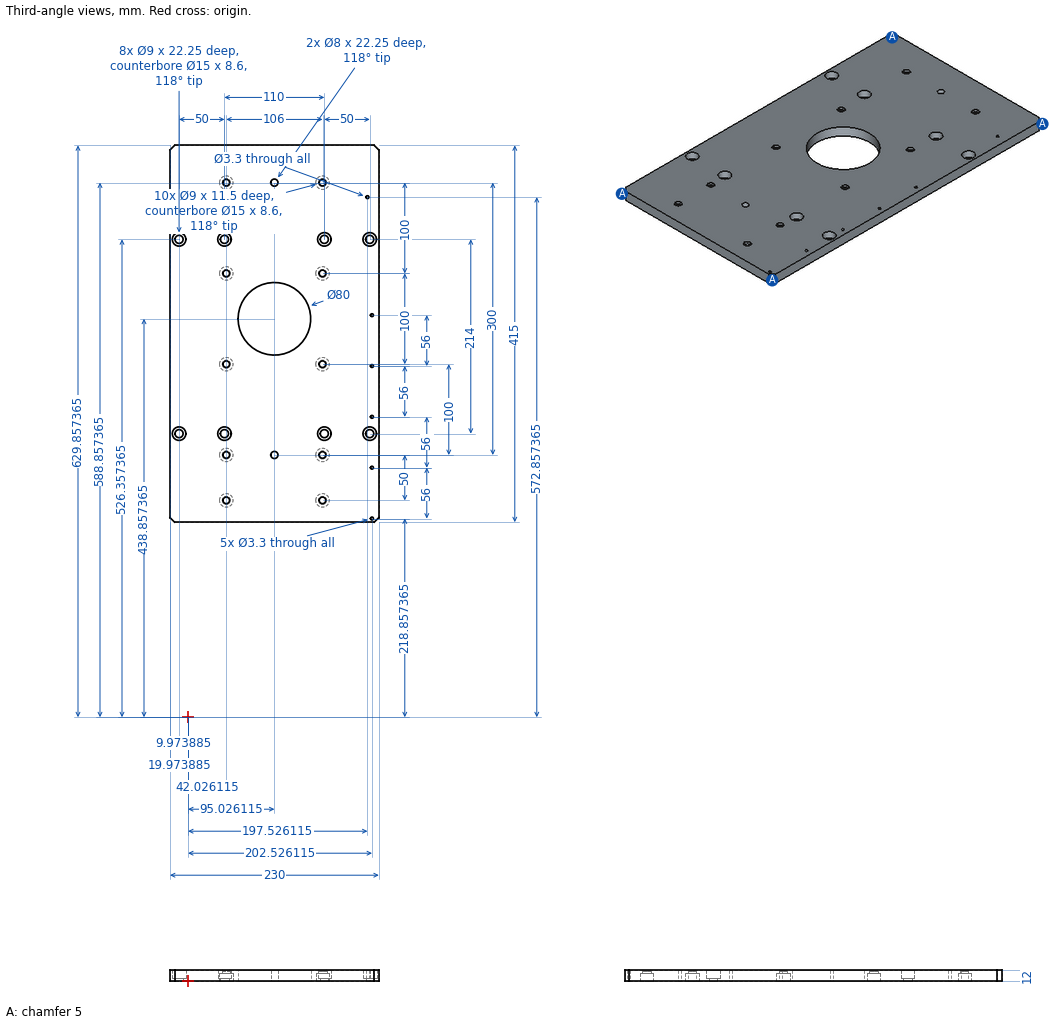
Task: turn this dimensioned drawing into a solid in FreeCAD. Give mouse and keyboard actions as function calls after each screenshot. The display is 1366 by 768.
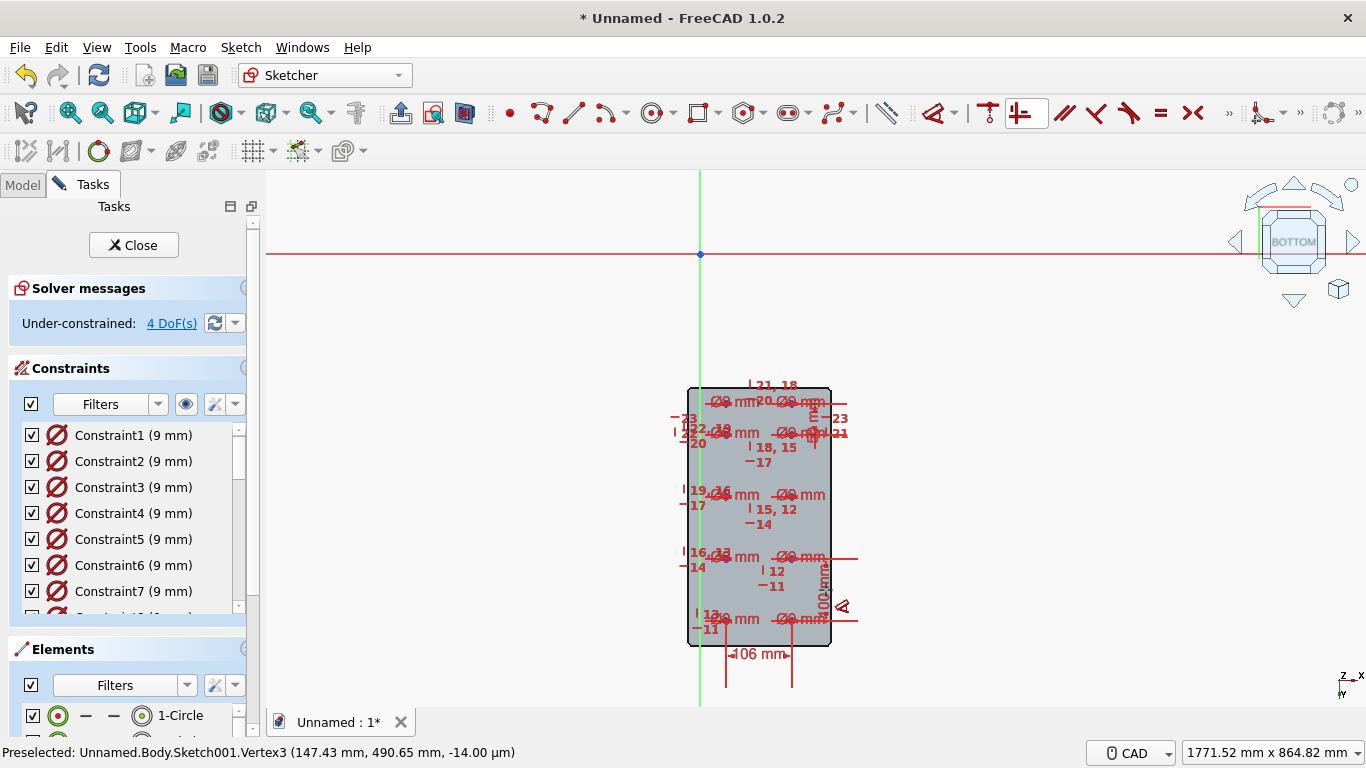
click(792, 559)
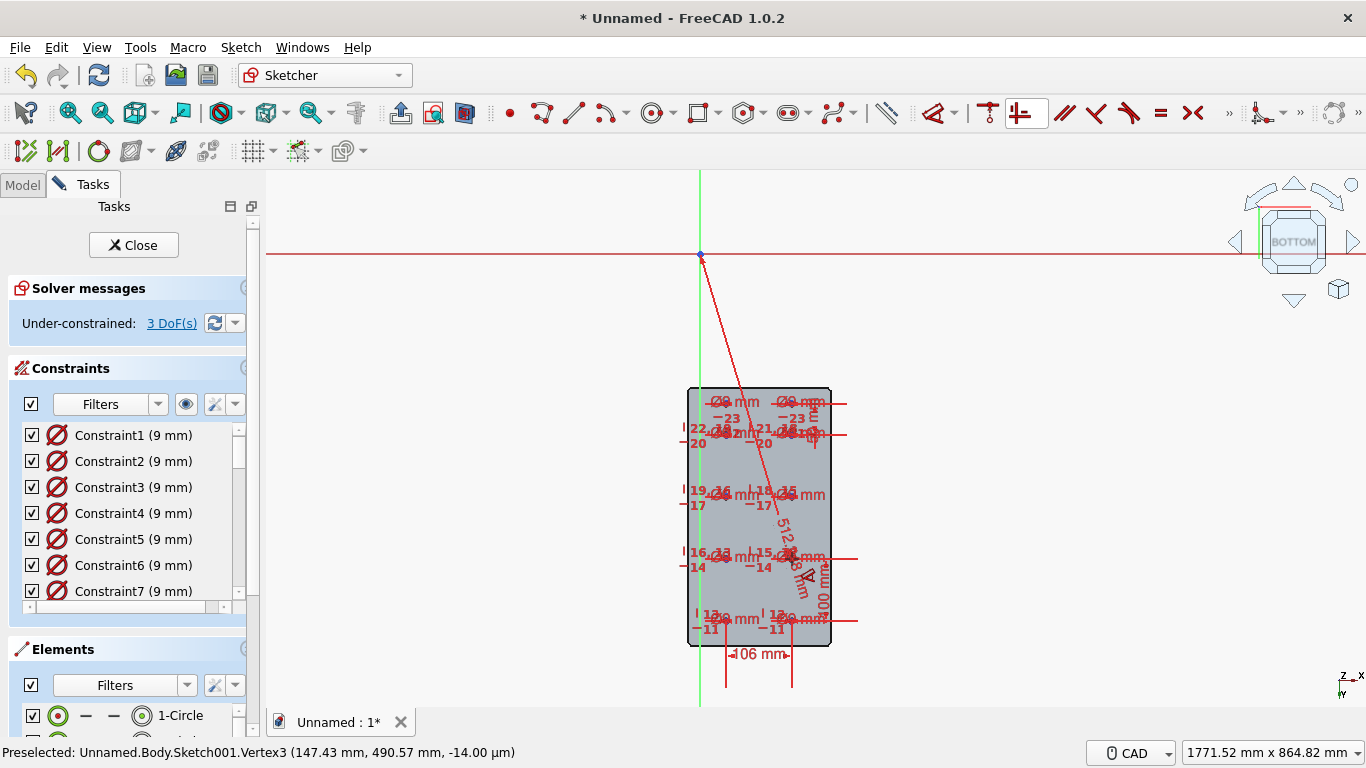
click(792, 497)
click(826, 528)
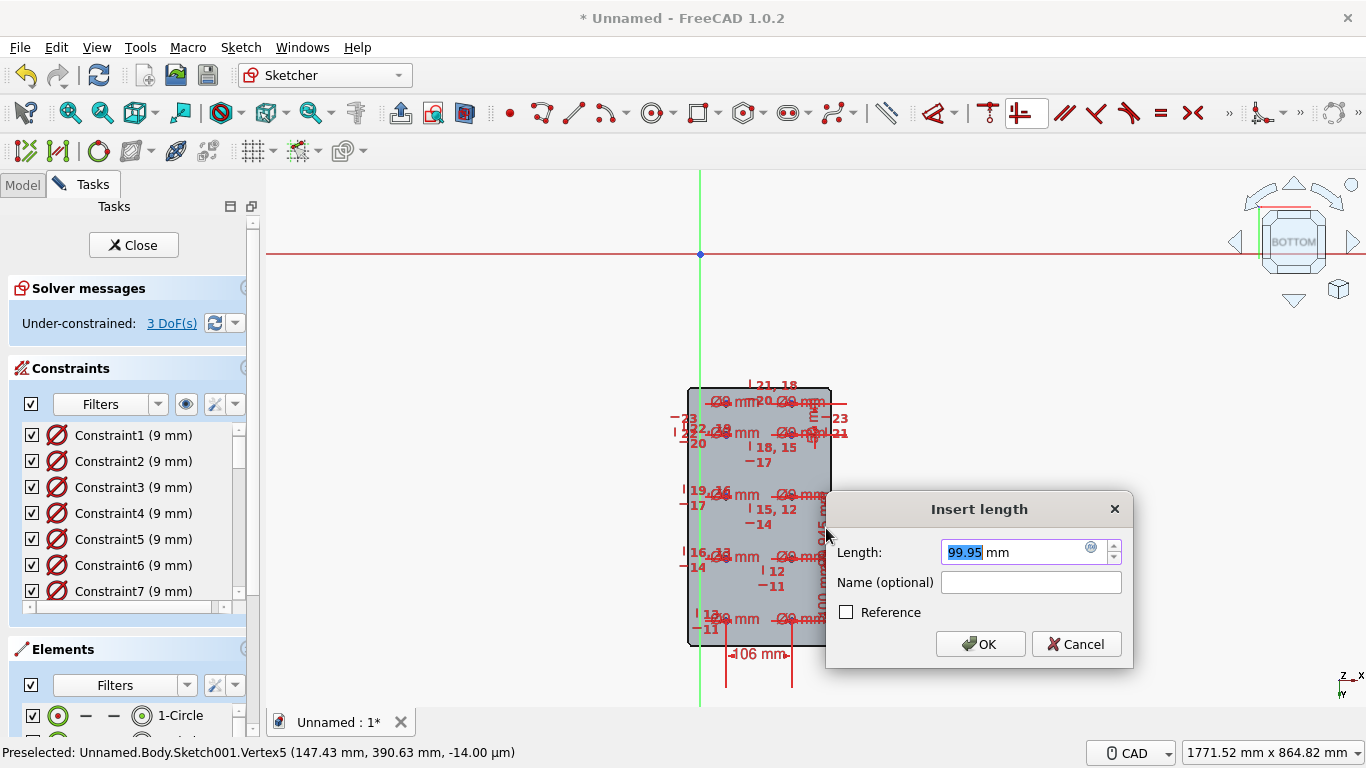
text(100)
key(Return)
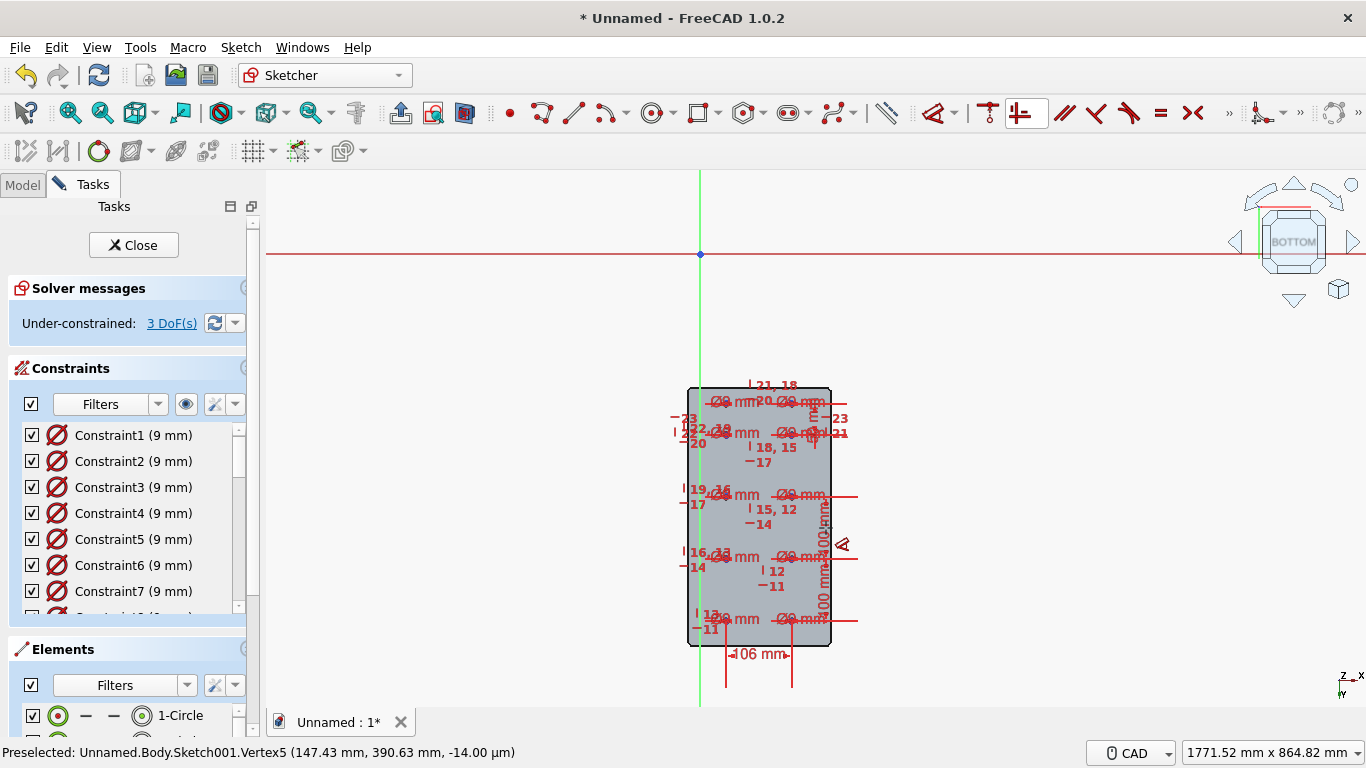
click(792, 497)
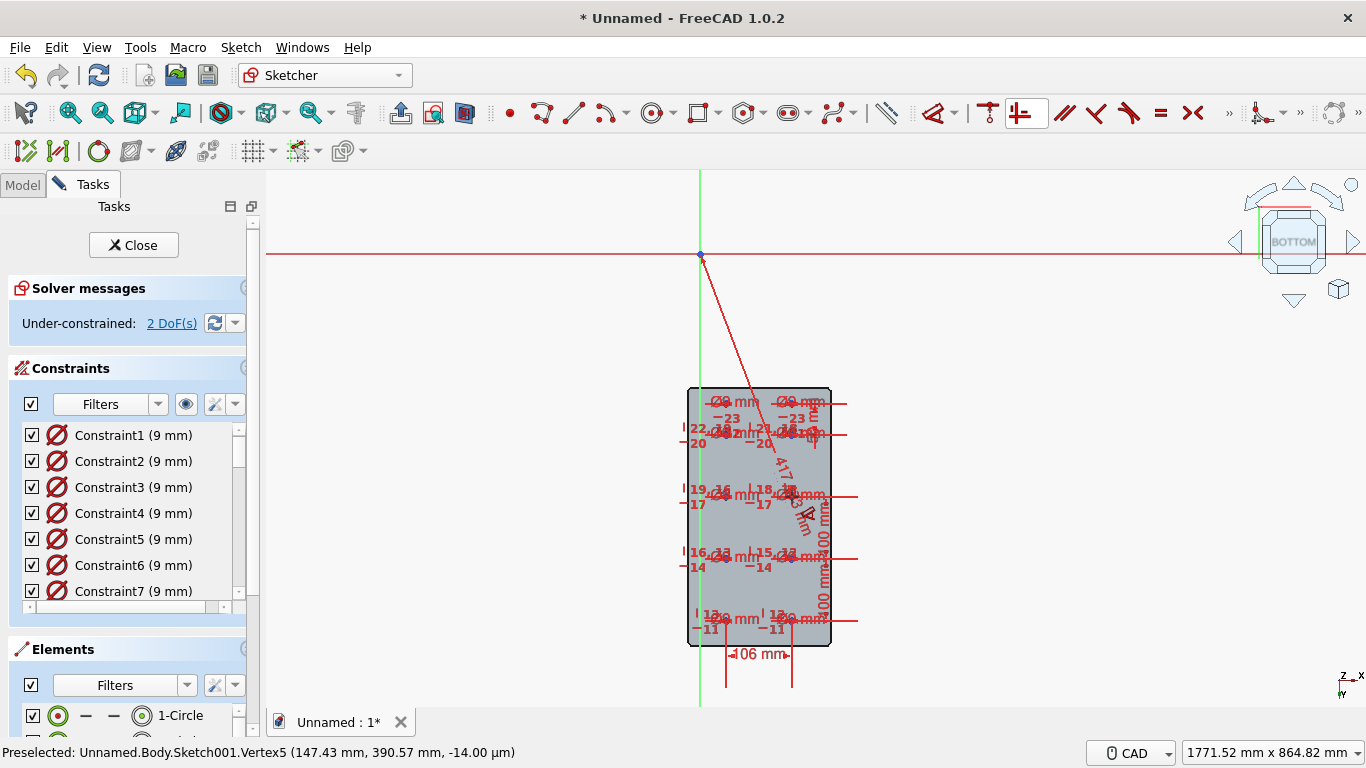
click(792, 435)
click(826, 466)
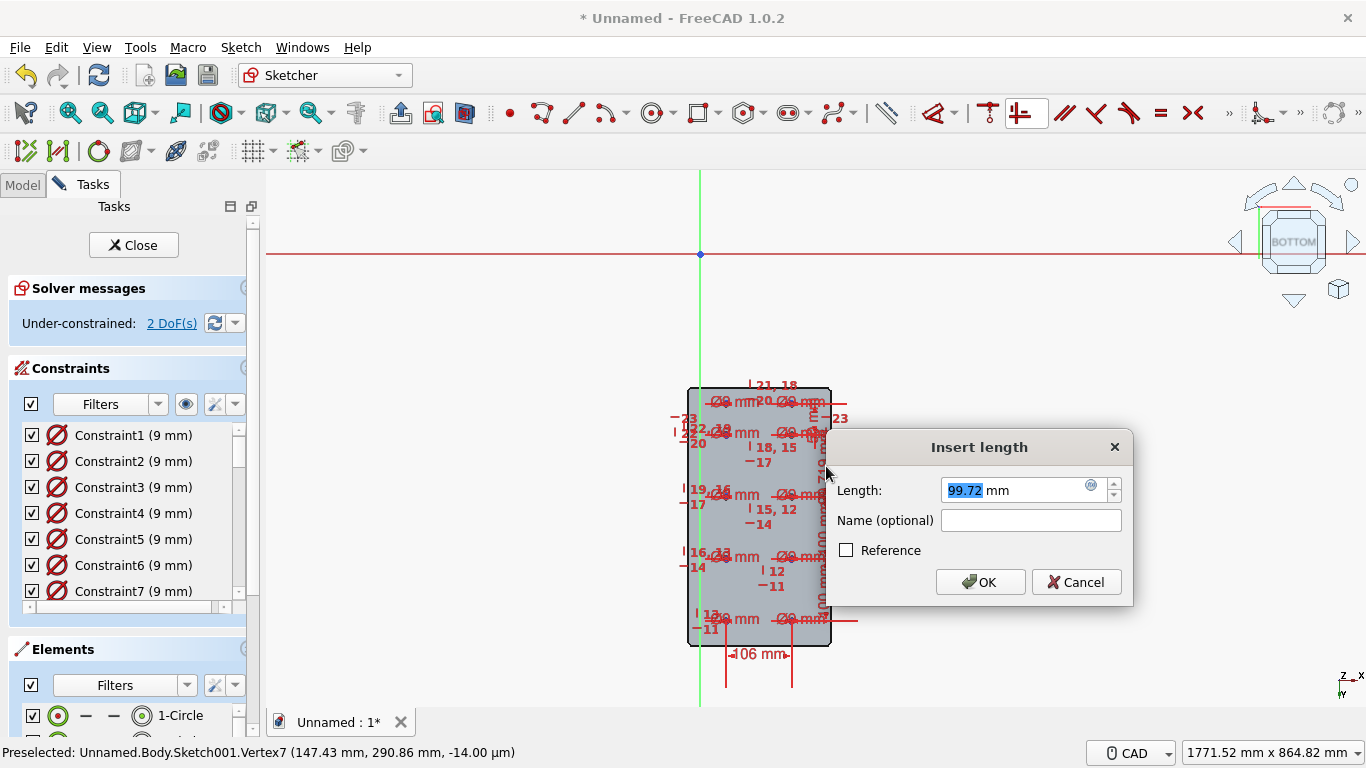
text(100)
key(Return)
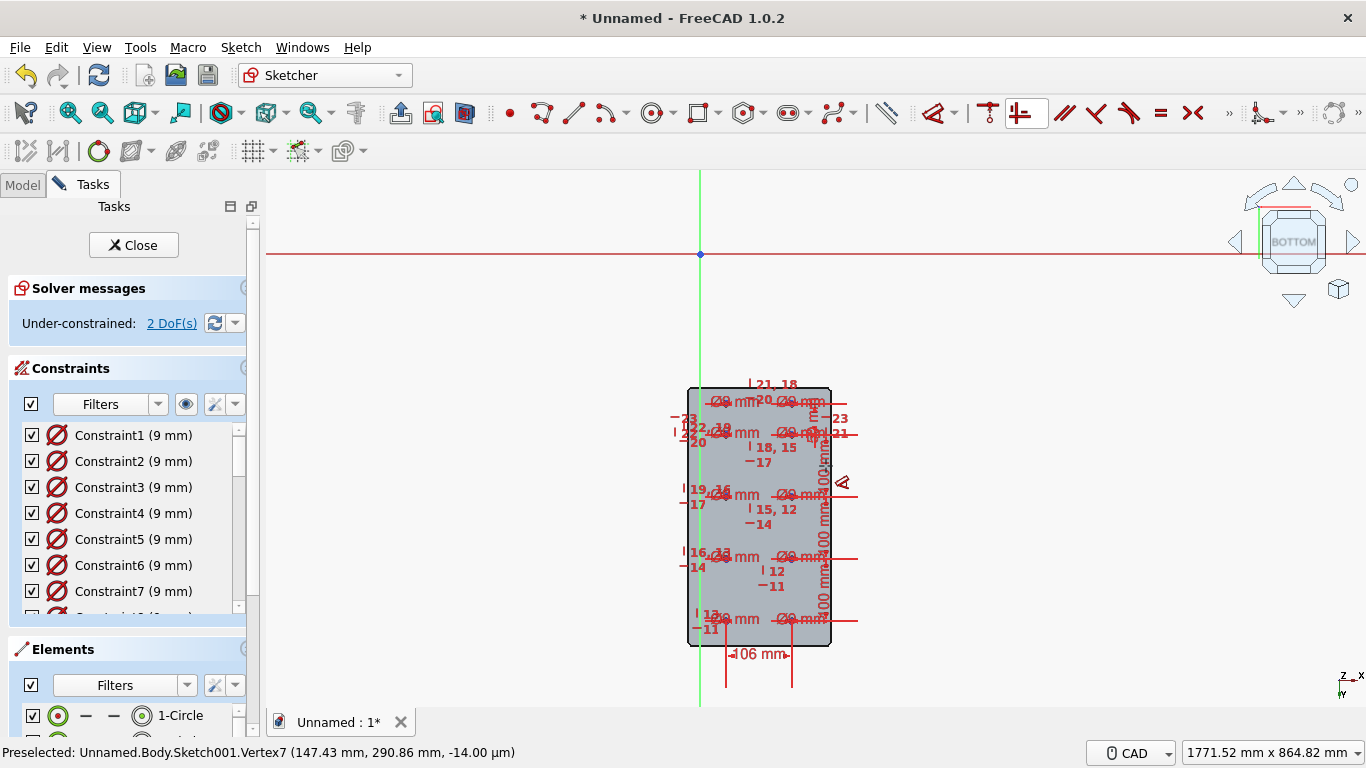
scroll(726, 621, up, 3)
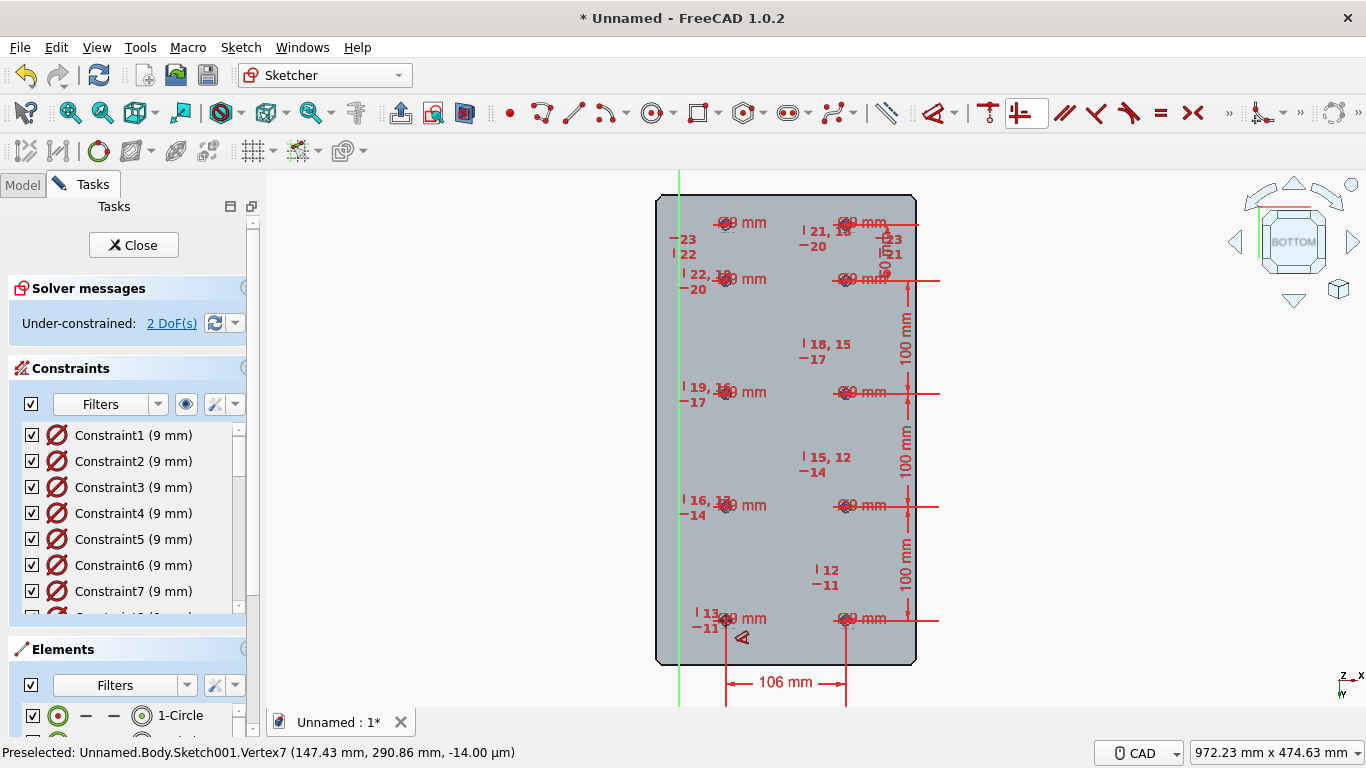
click(726, 621)
click(702, 655)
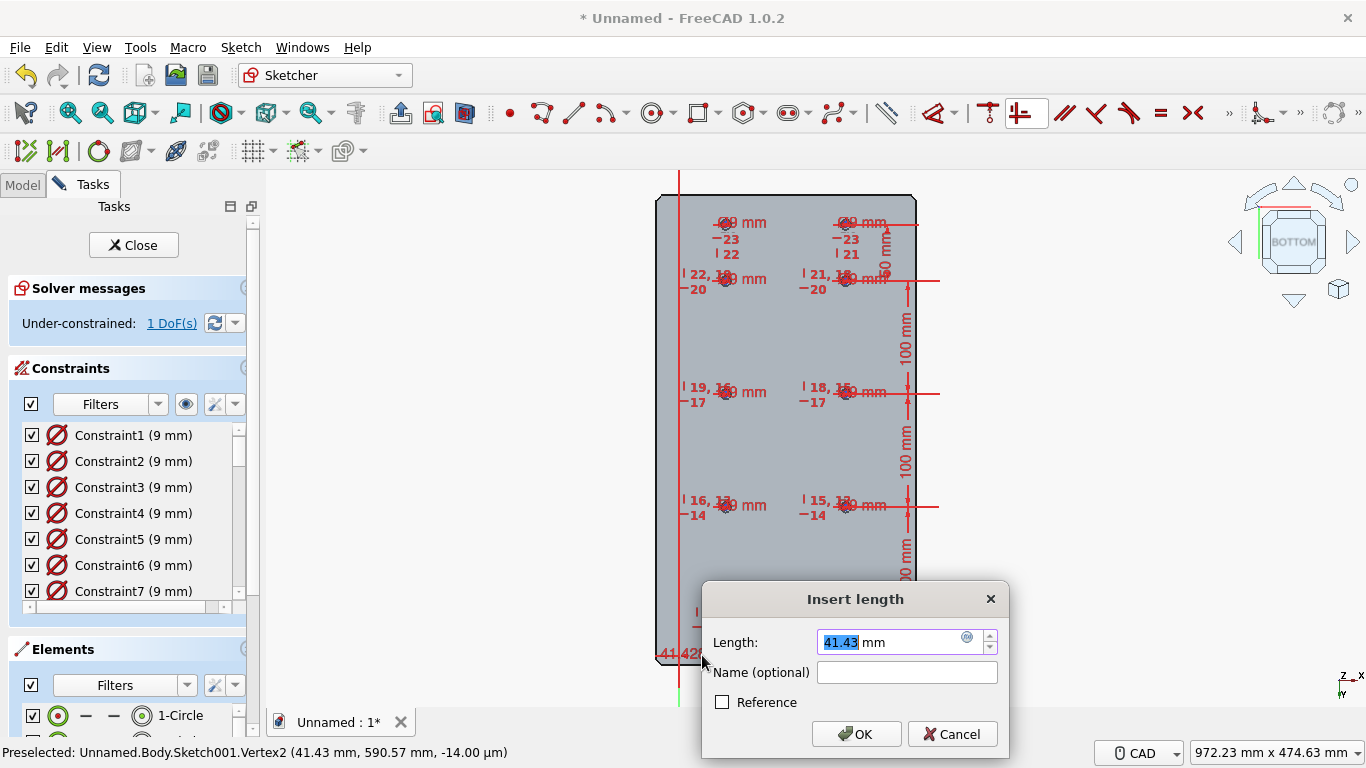
text(42.026115)
key(Return)